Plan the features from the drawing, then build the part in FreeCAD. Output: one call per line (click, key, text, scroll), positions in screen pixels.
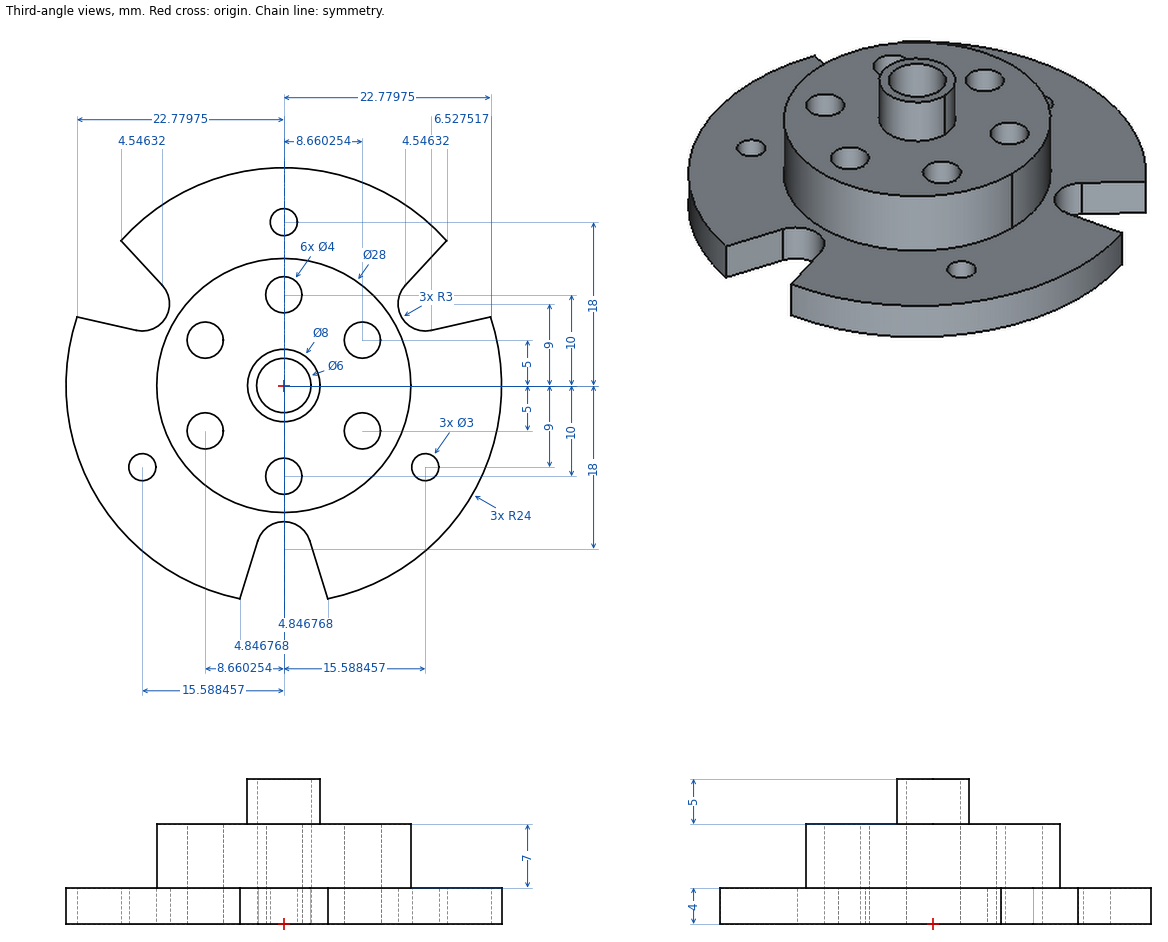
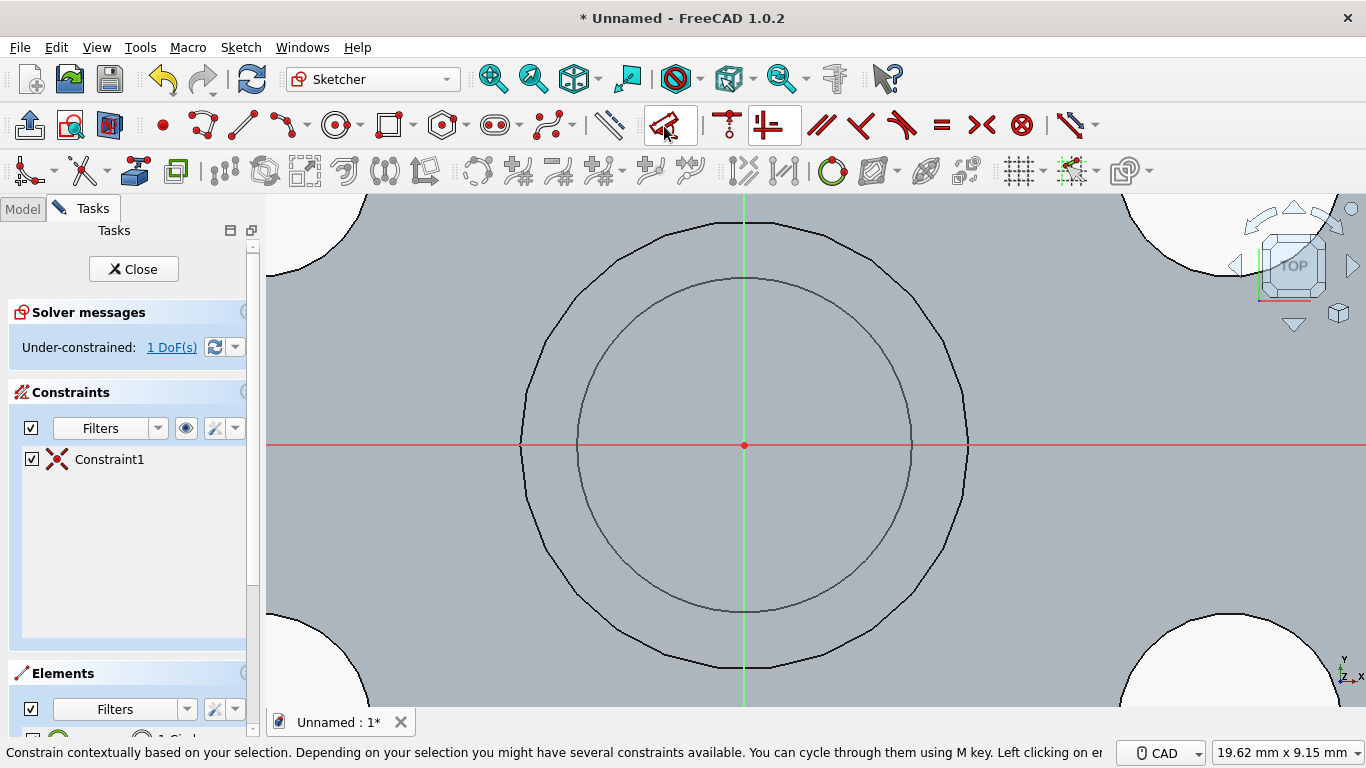
click(862, 326)
click(884, 303)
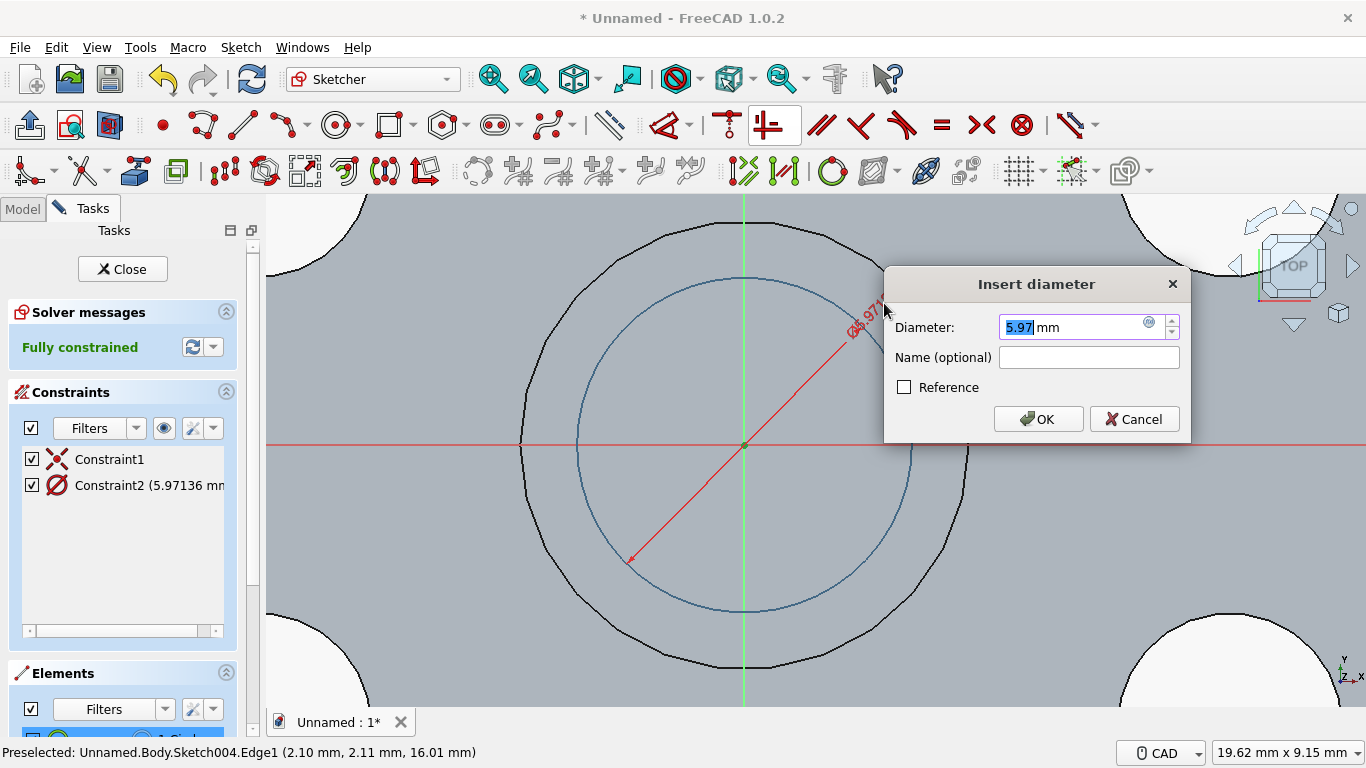
text(6)
key(Return)
key(Escape)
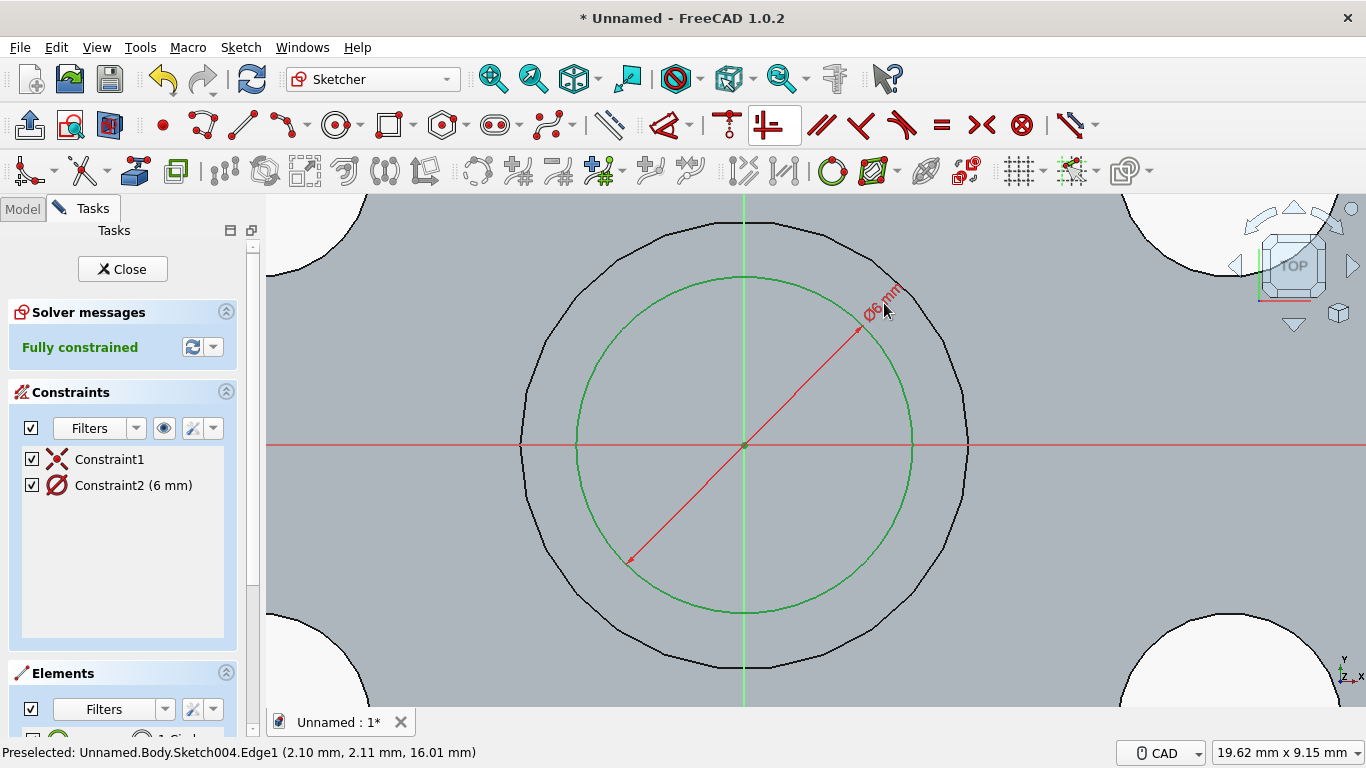
click(123, 269)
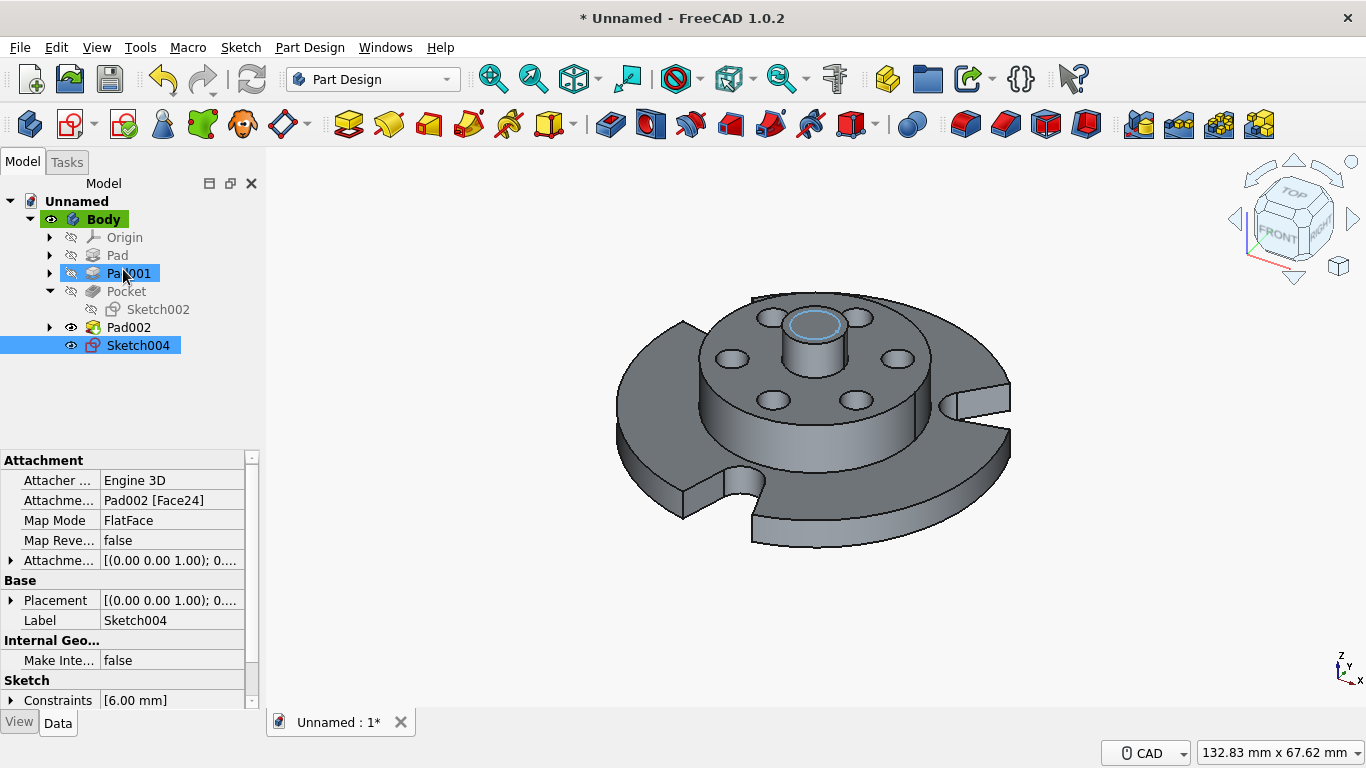
click(612, 124)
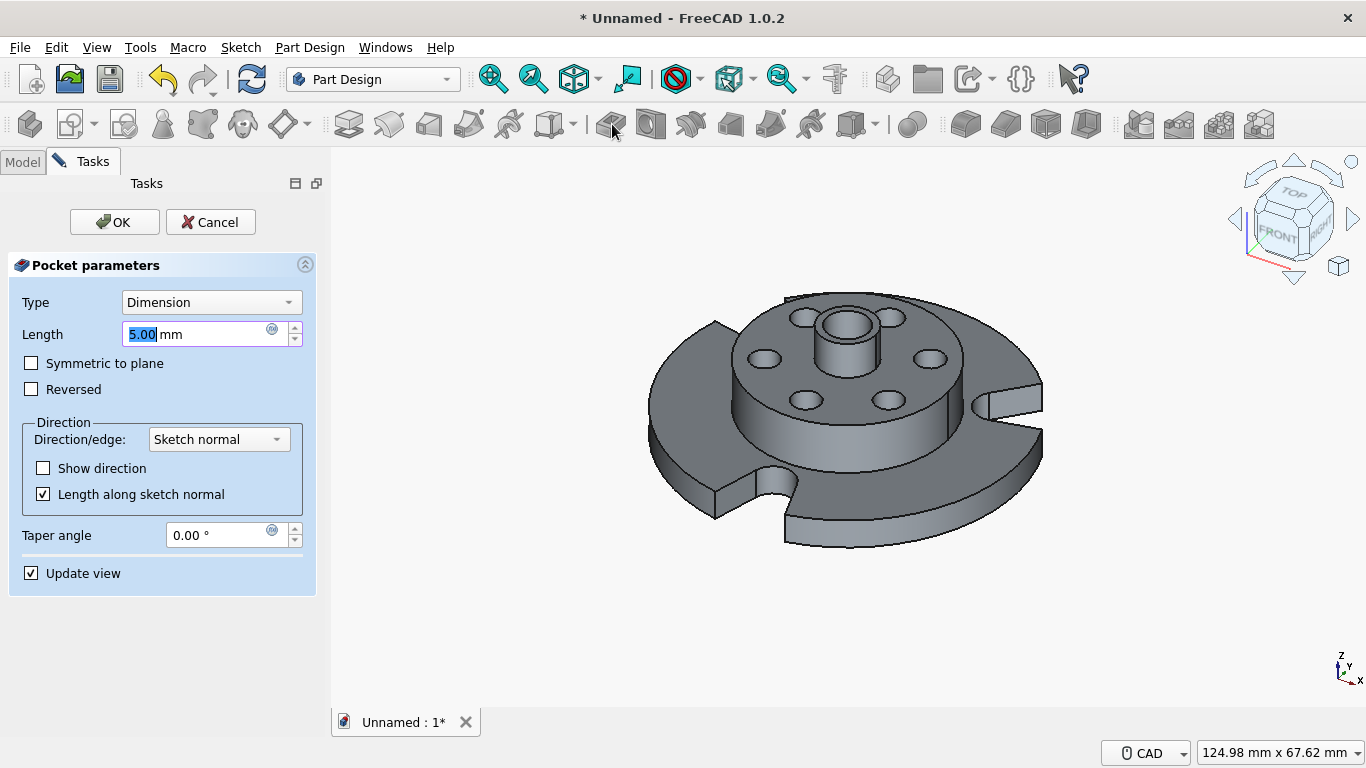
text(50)
key(Tab)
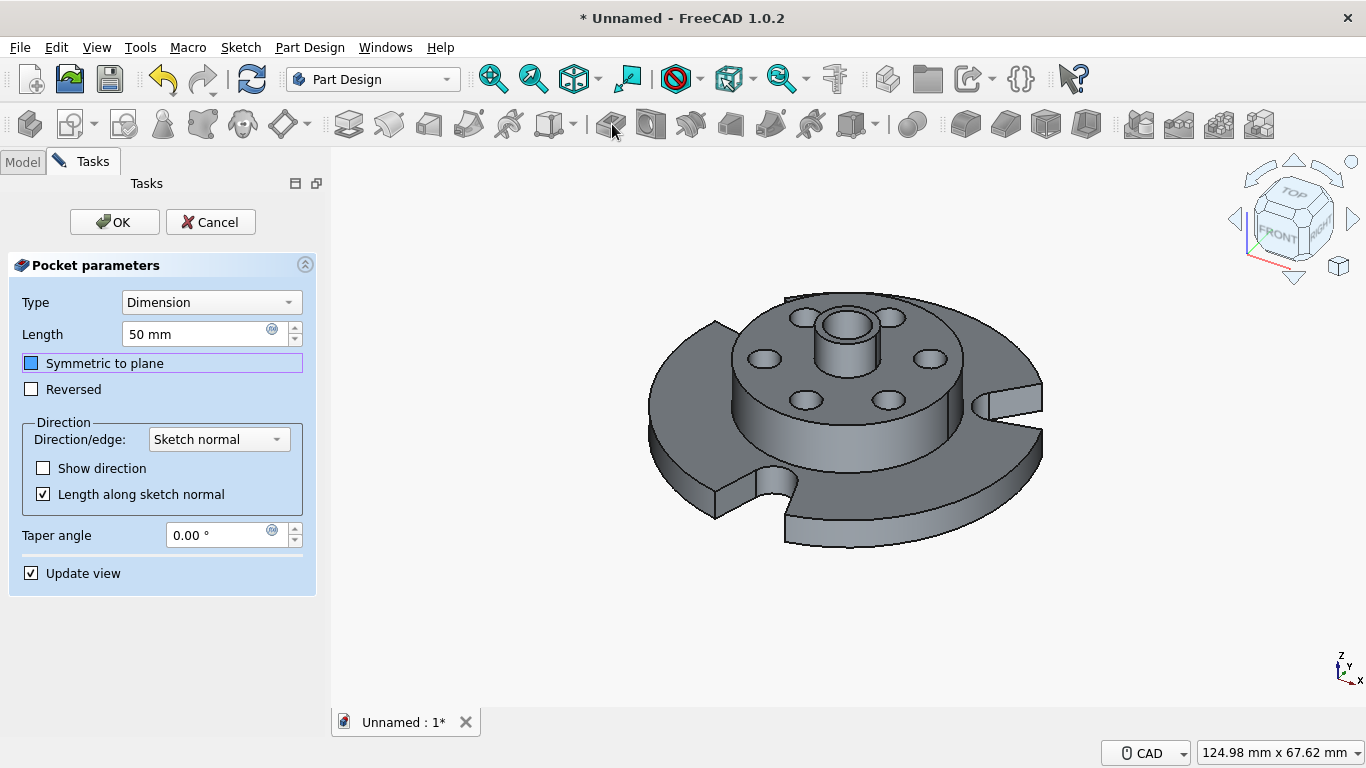
click(115, 222)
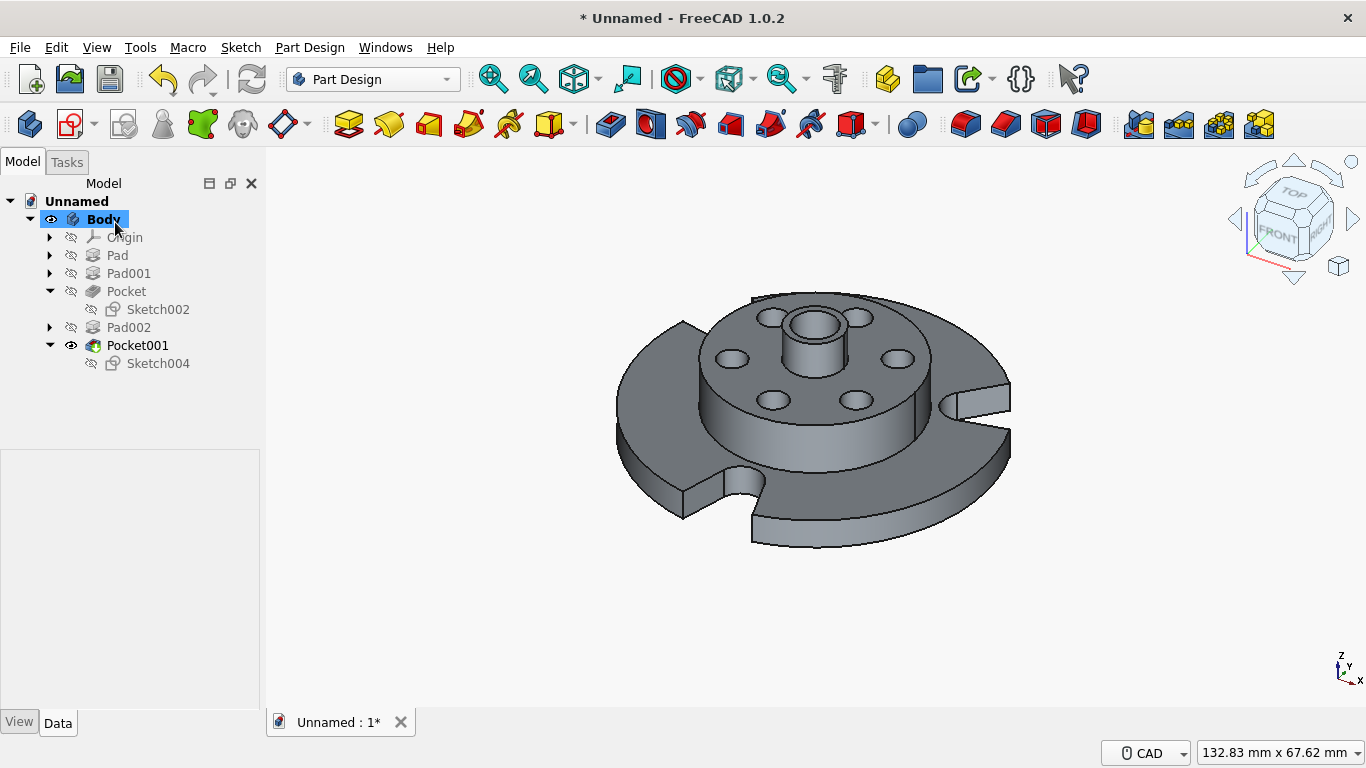
click(858, 493)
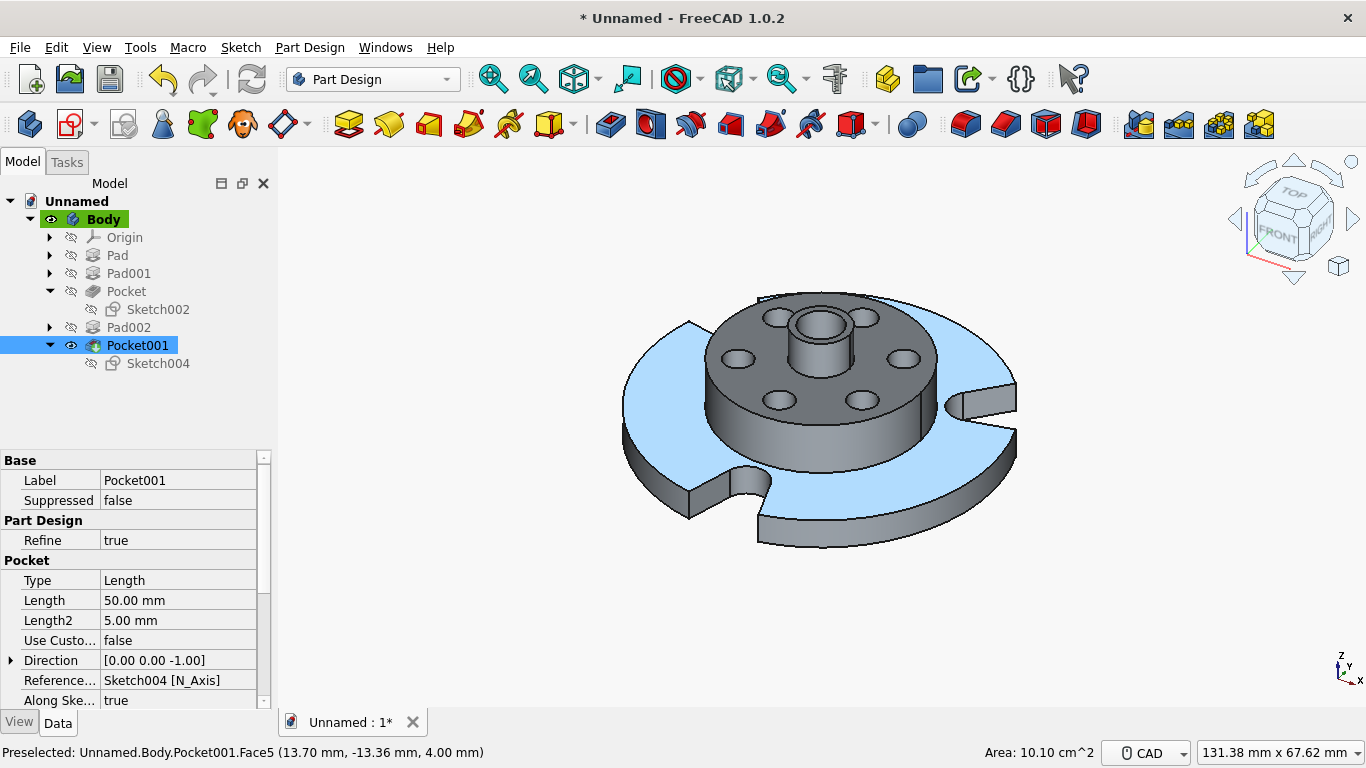
click(70, 124)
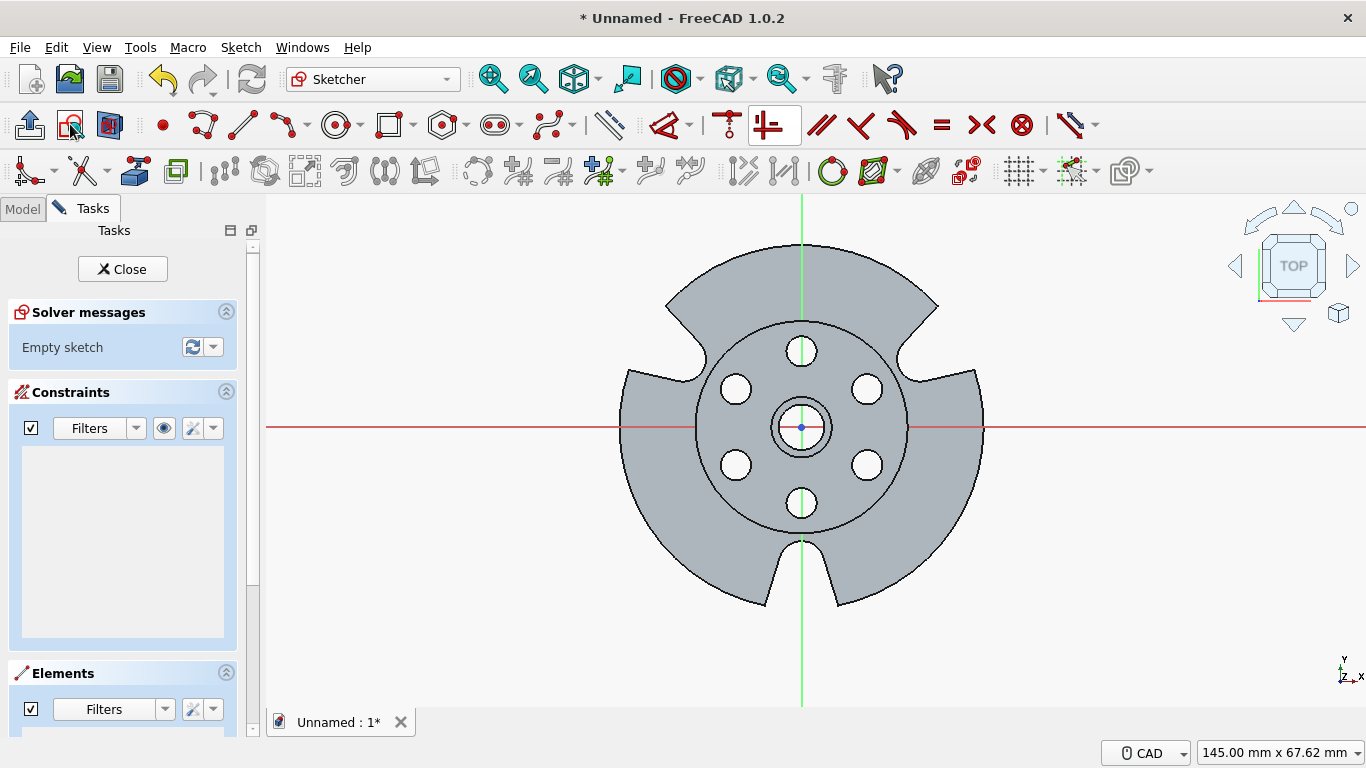
scroll(911, 276, up, 2)